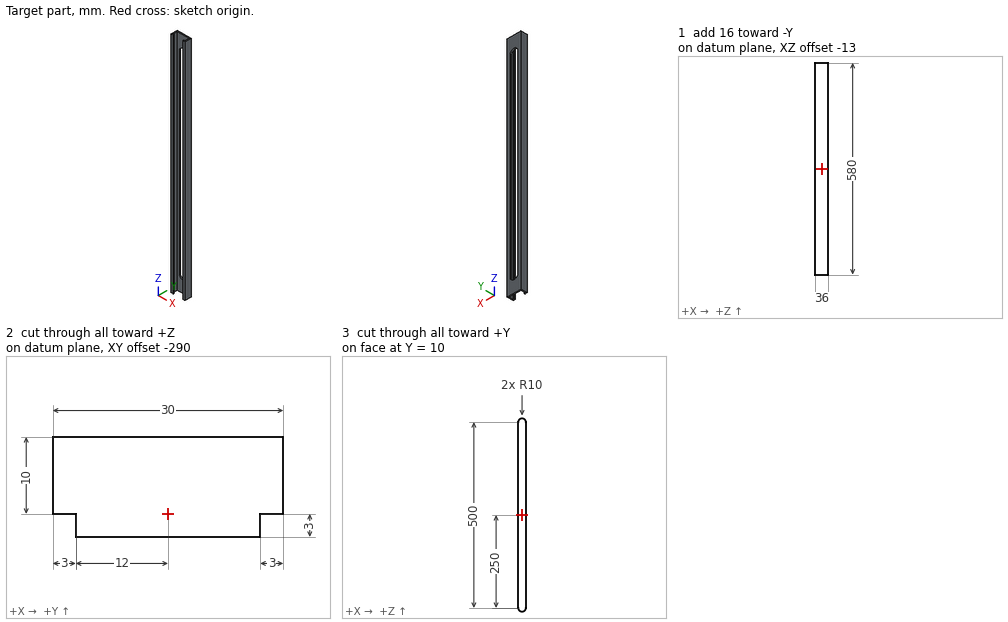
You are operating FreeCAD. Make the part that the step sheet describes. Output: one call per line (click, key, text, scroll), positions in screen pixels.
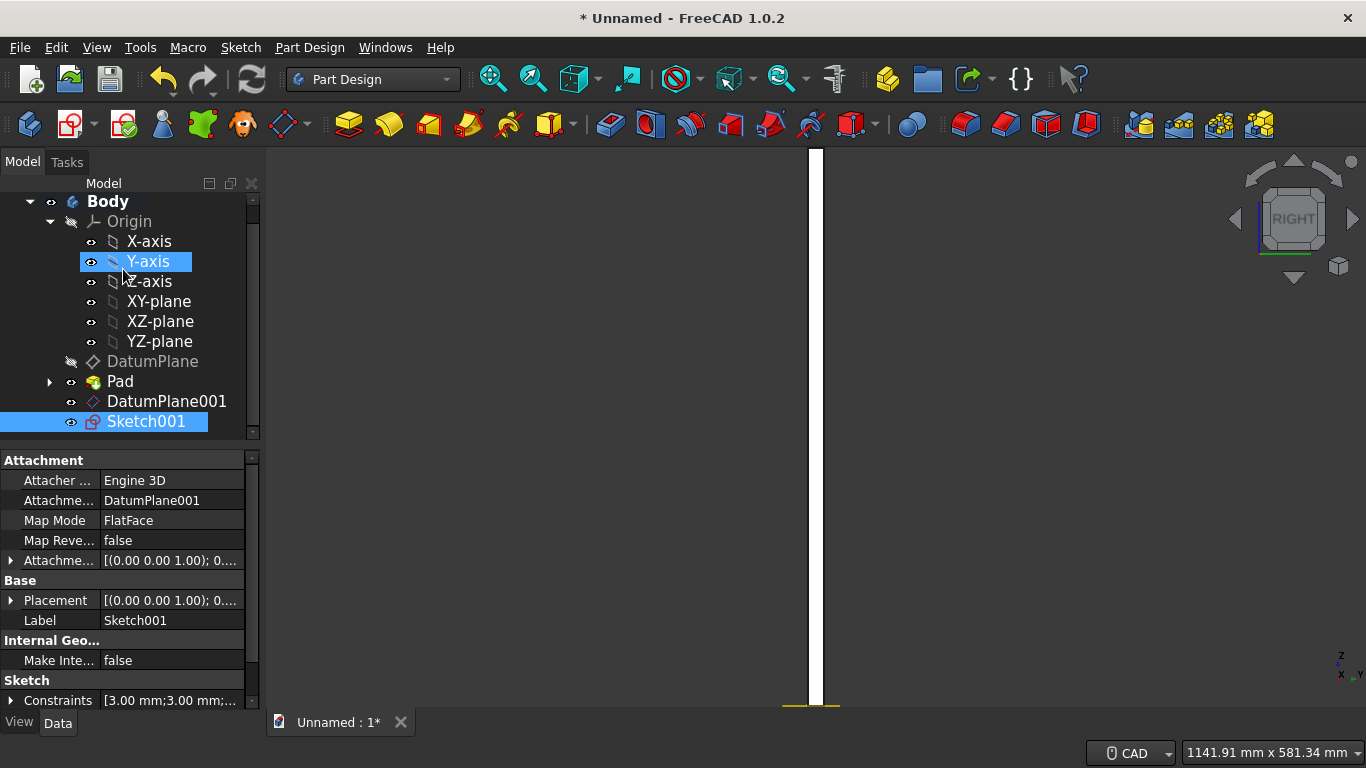
click(612, 124)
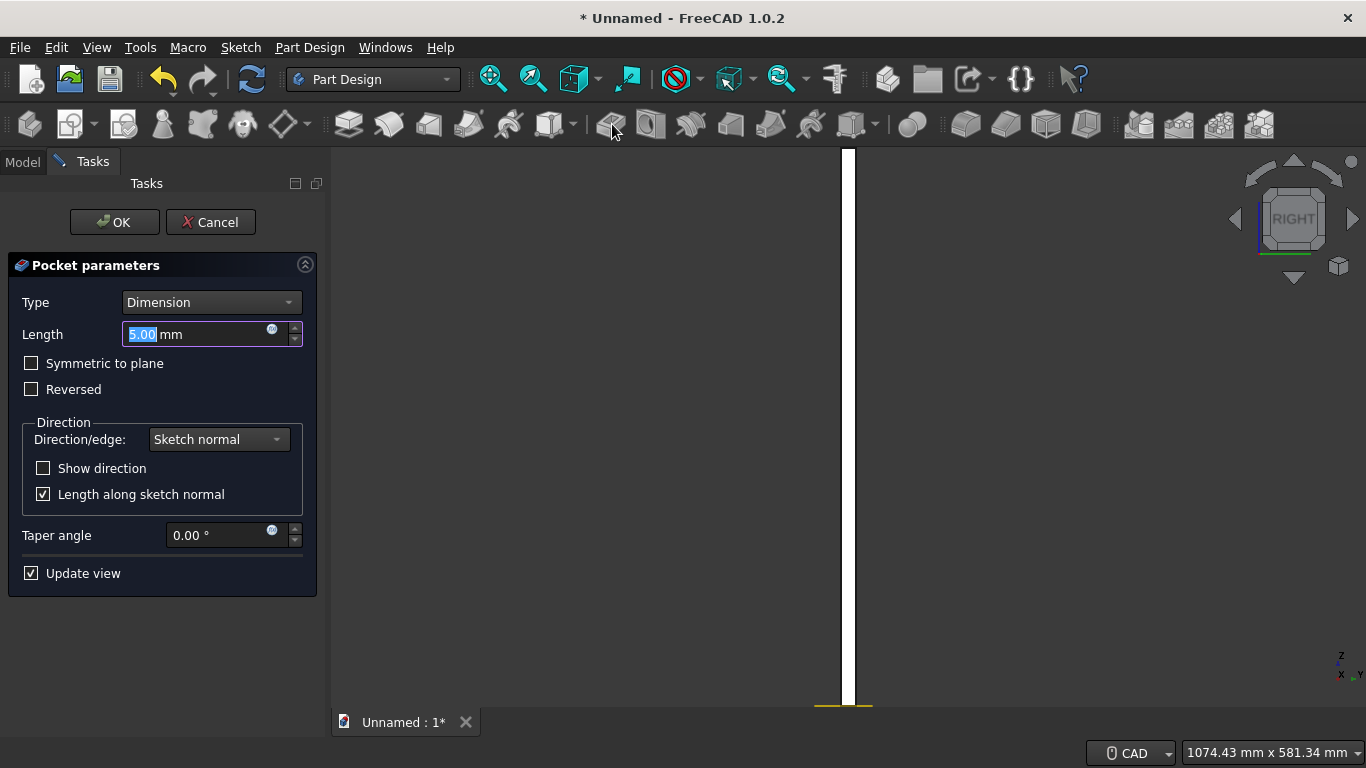
click(212, 302)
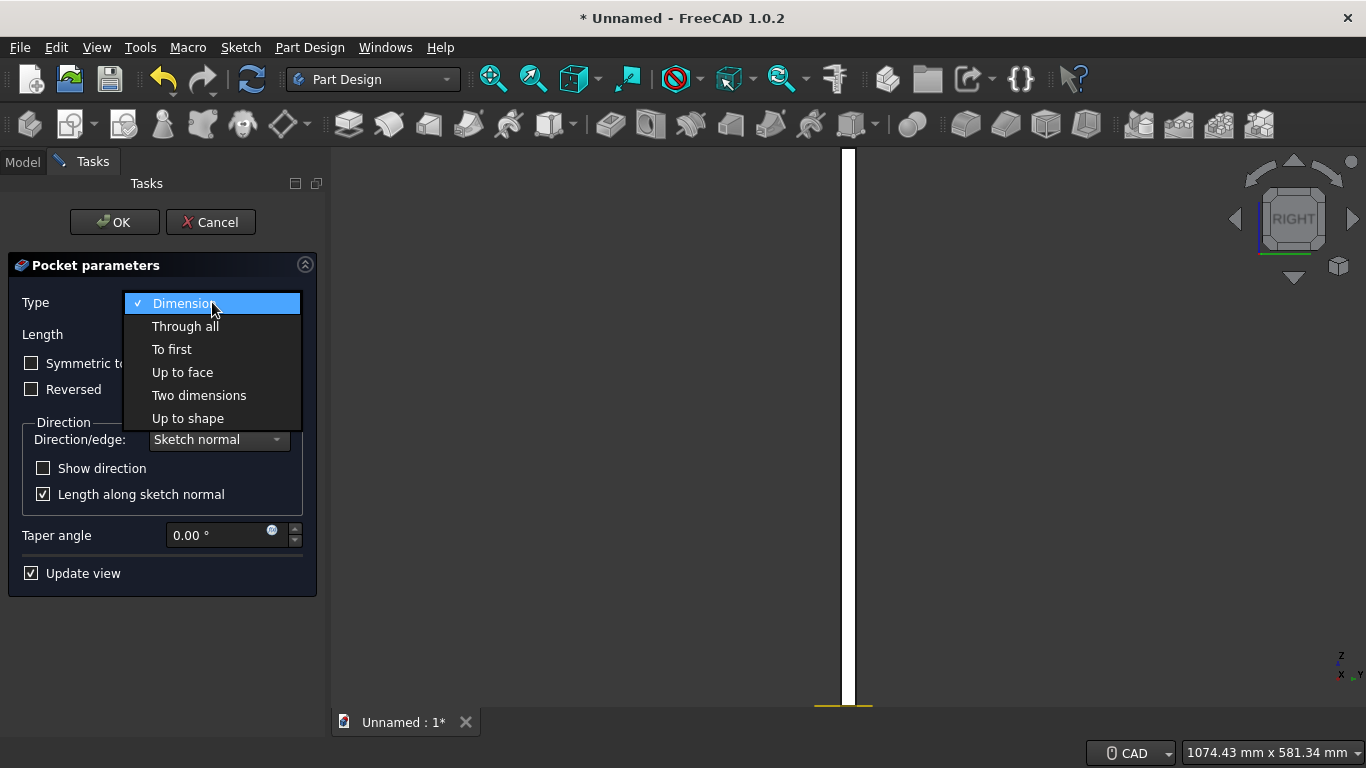
click(212, 326)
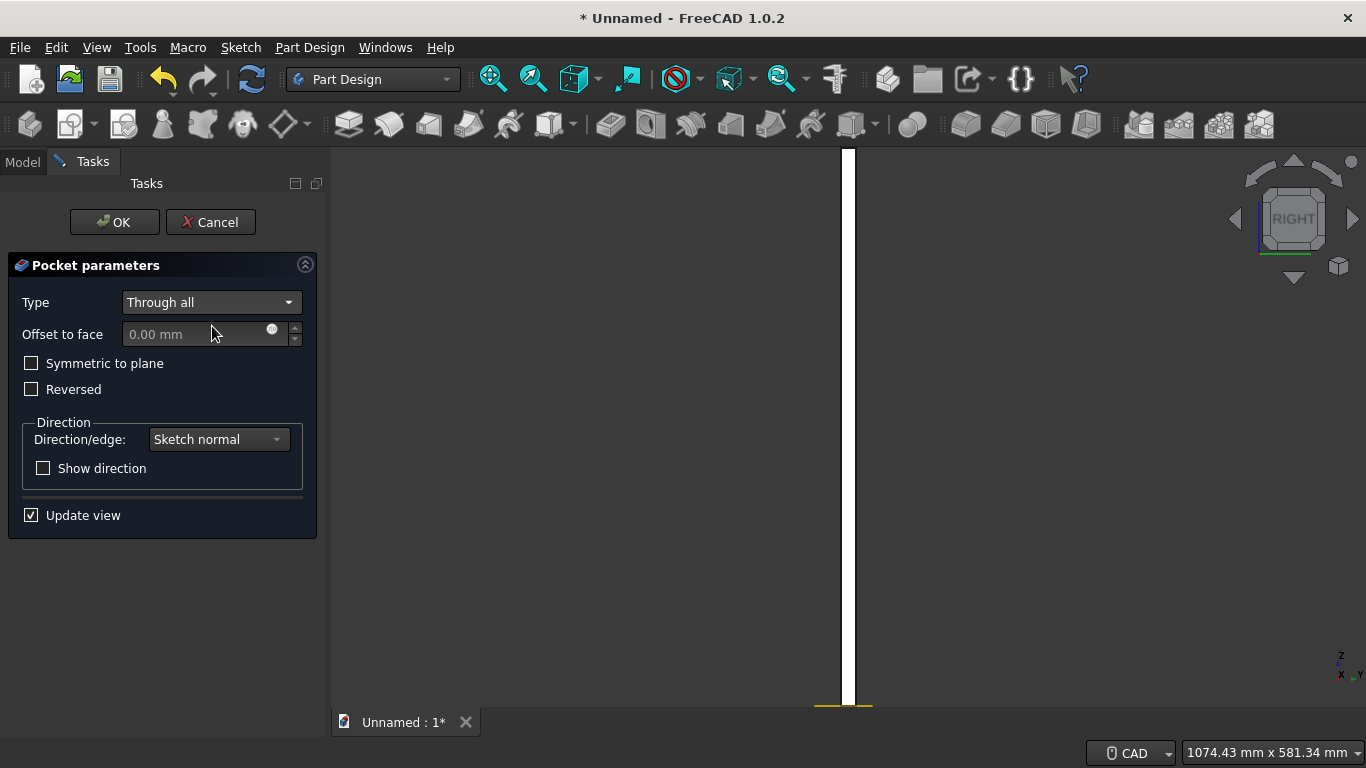
click(30, 389)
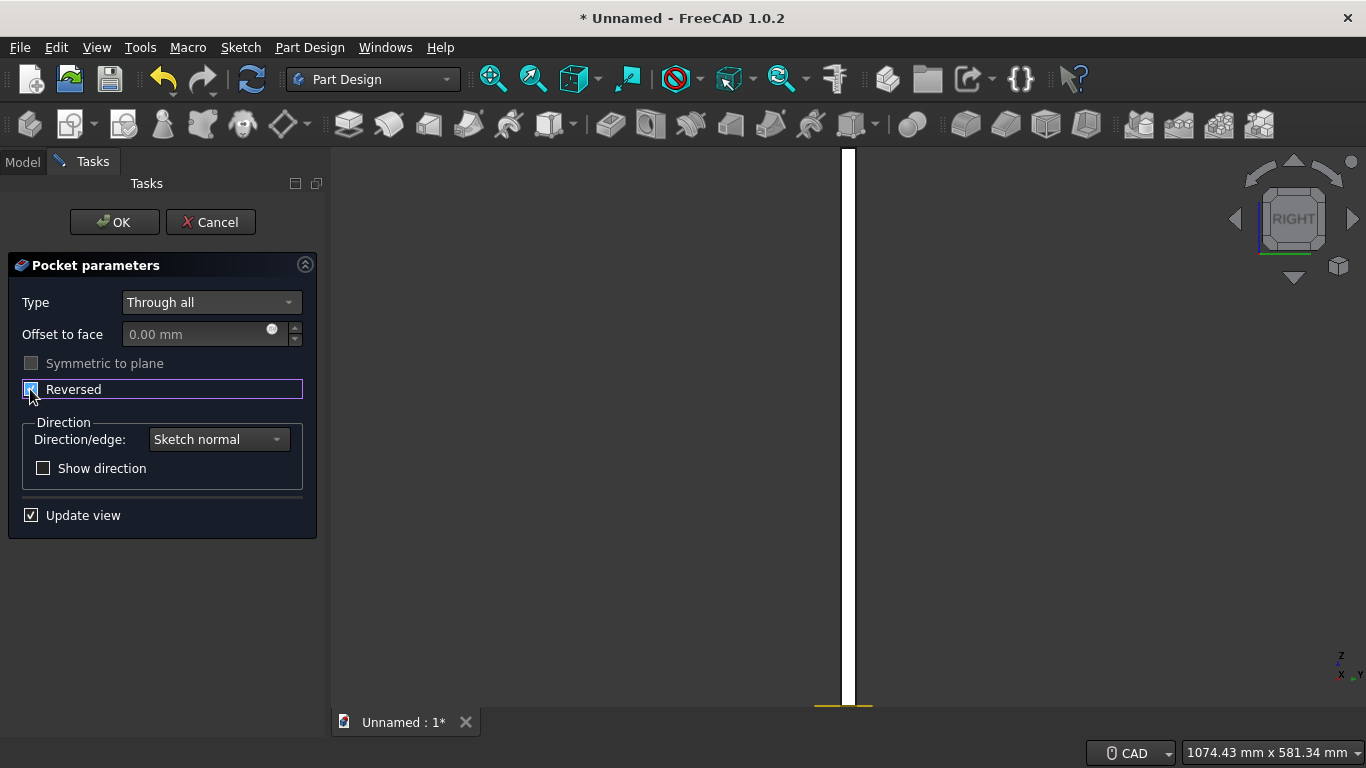
click(115, 222)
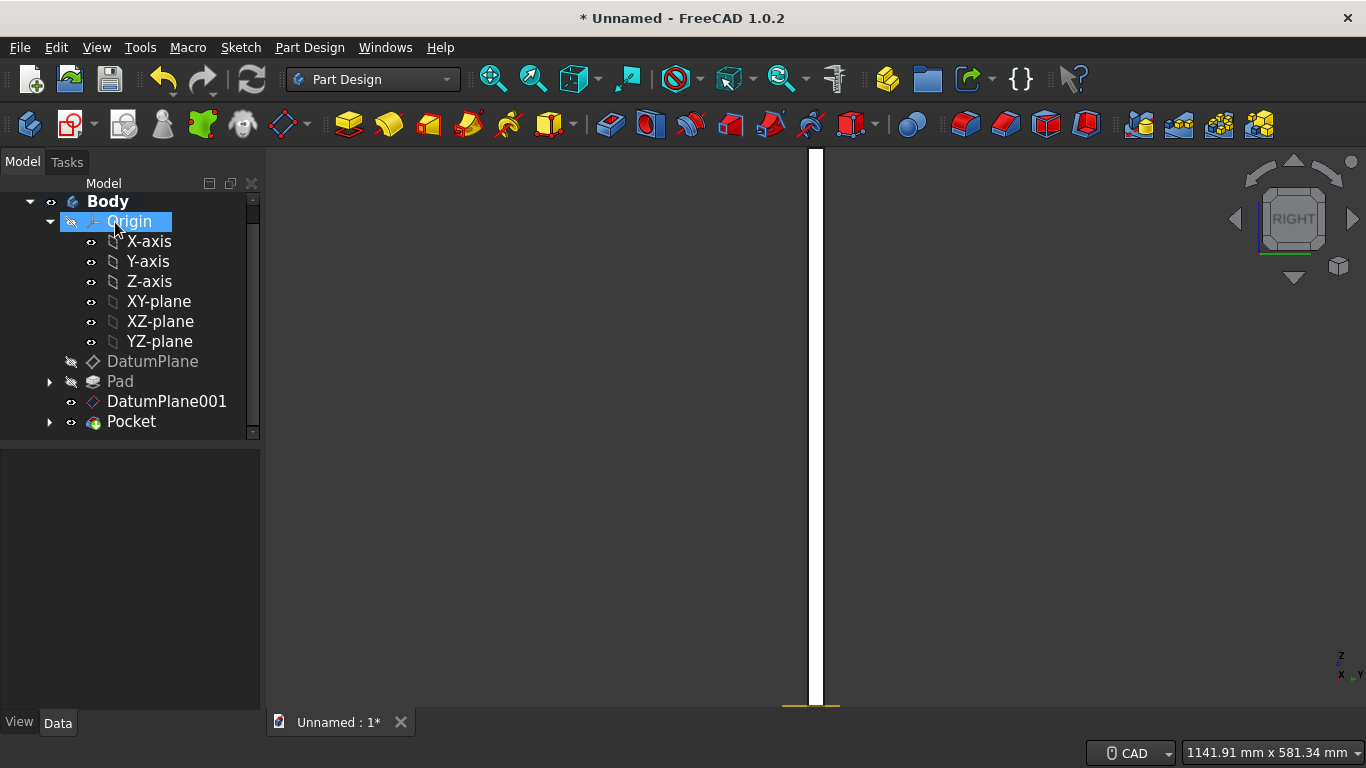
click(116, 402)
key(space)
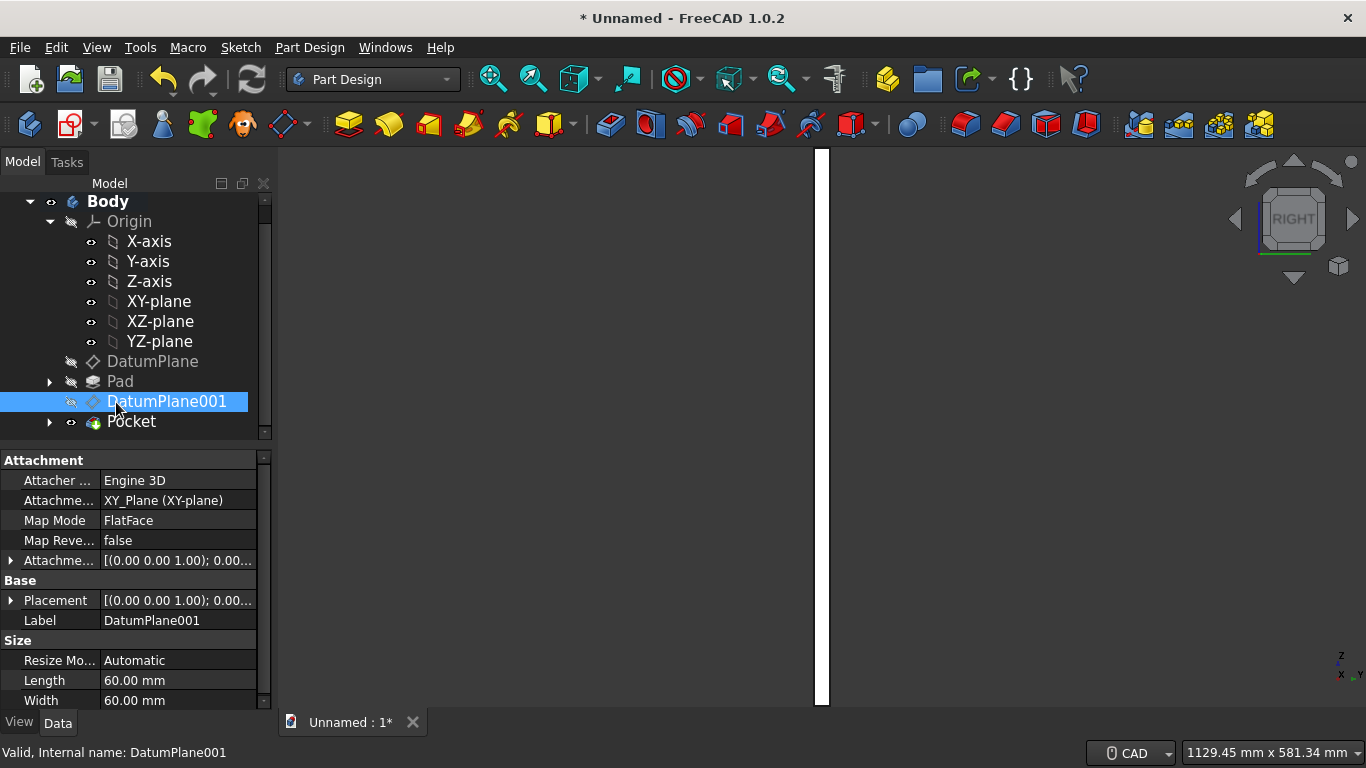
key(0)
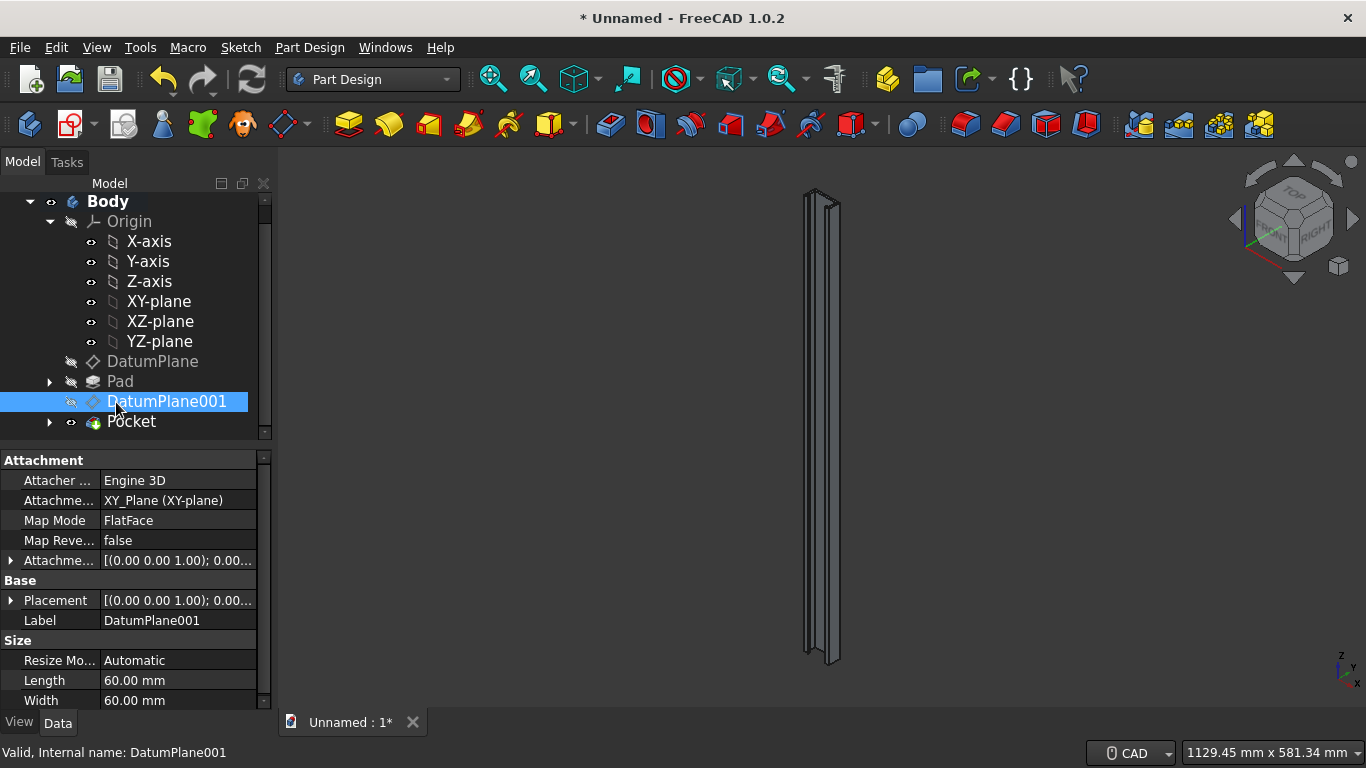
key(1)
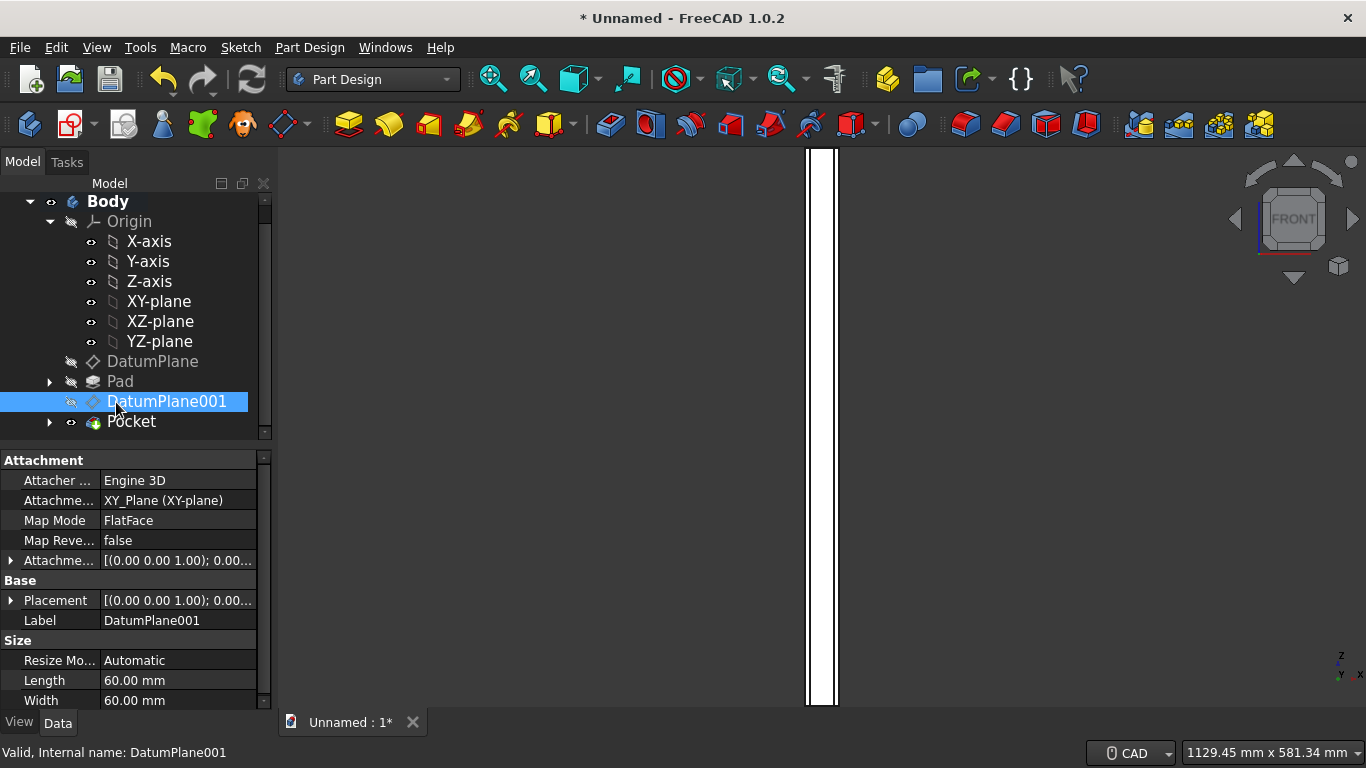
click(822, 187)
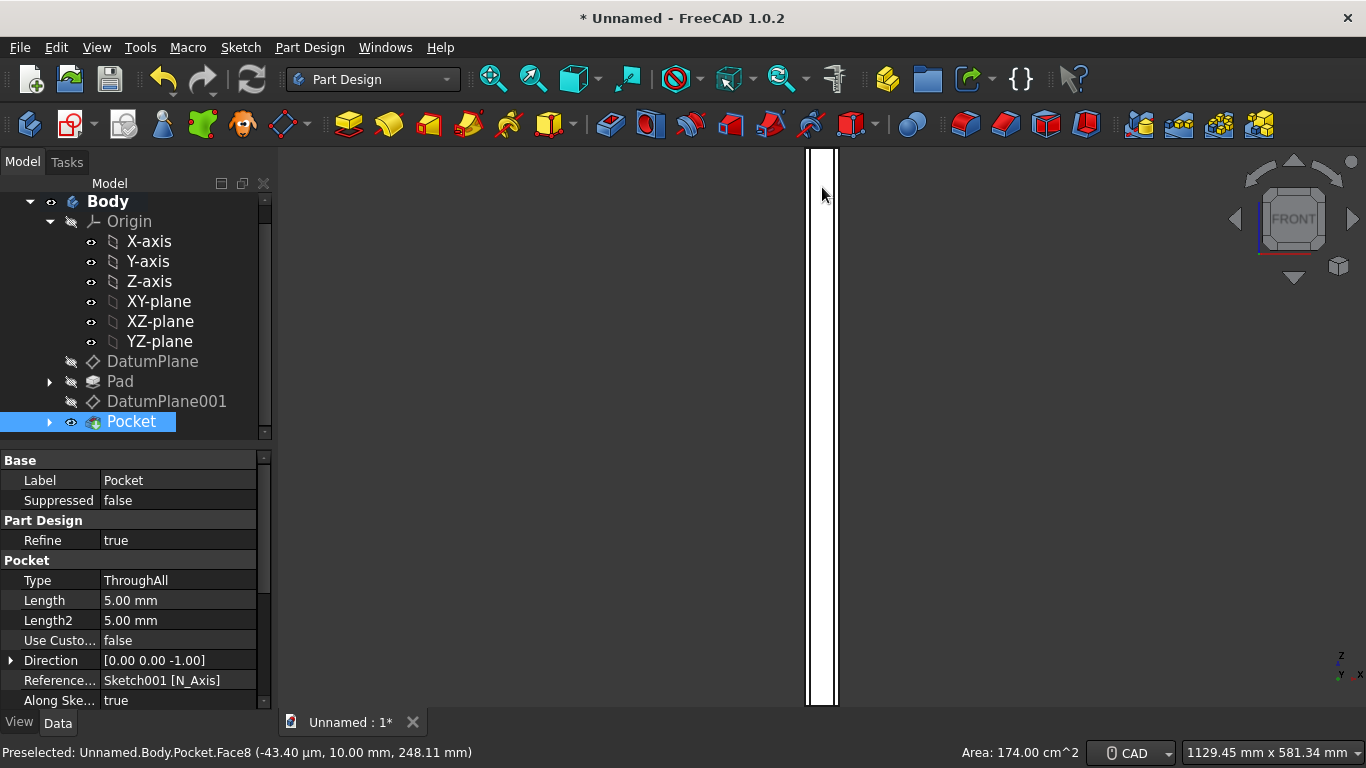
click(70, 124)